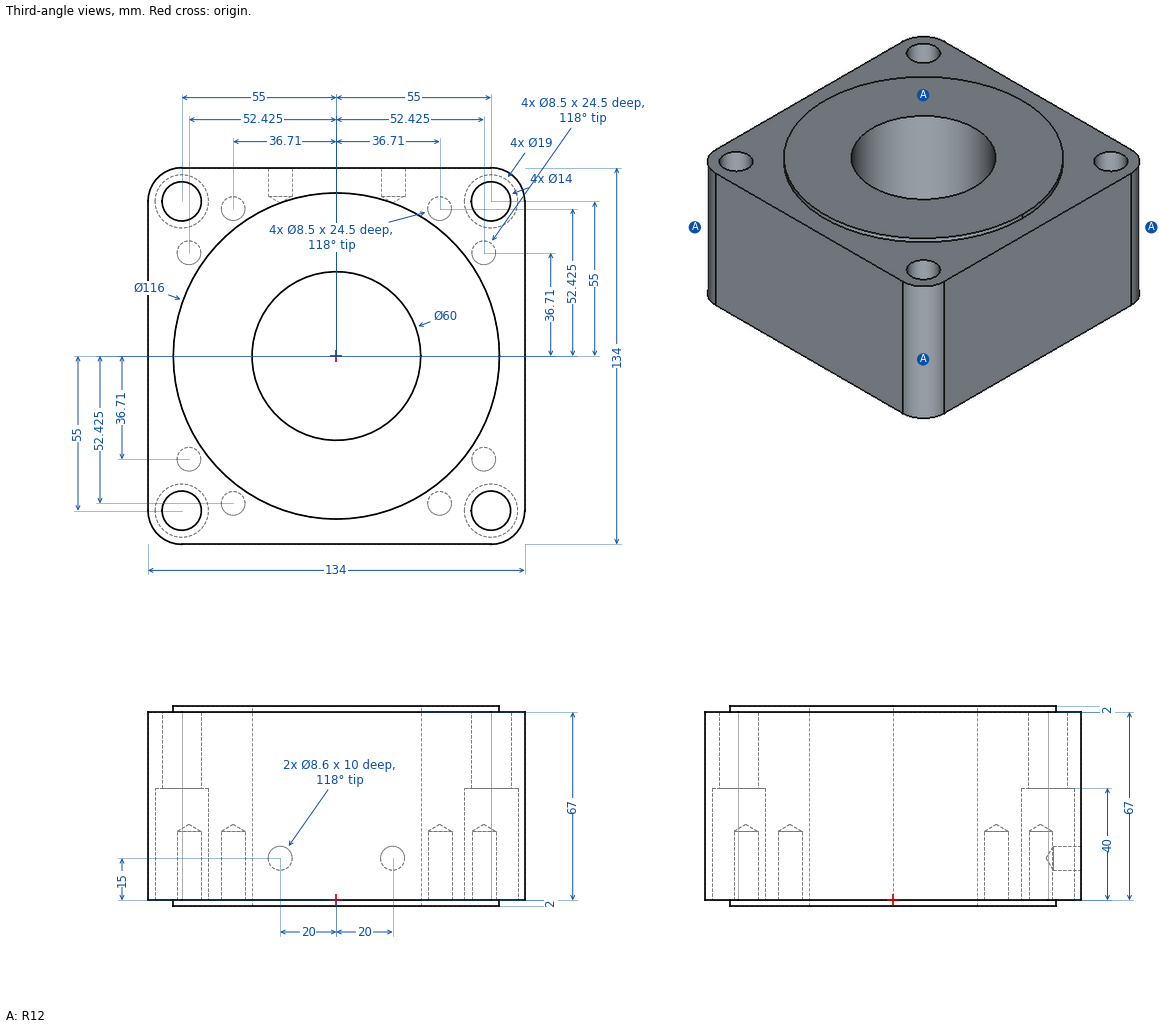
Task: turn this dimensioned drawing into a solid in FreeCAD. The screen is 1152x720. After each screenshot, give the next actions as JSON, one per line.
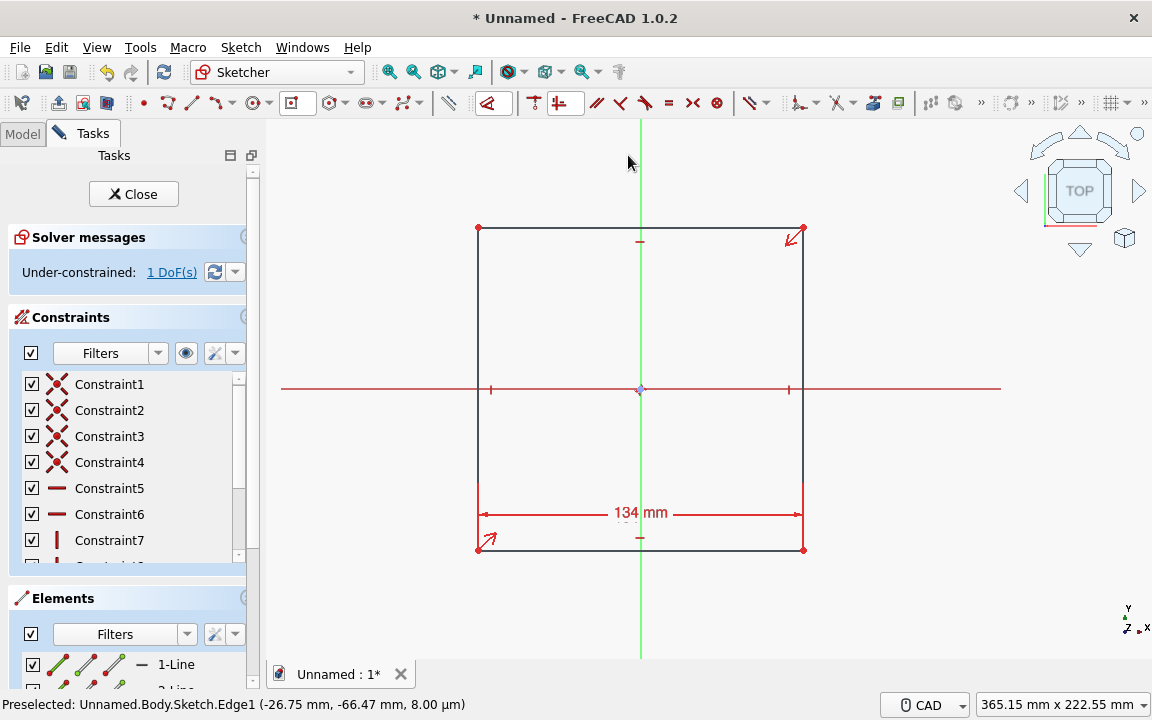
{"action": "left_click", "coordinate": [803, 454]}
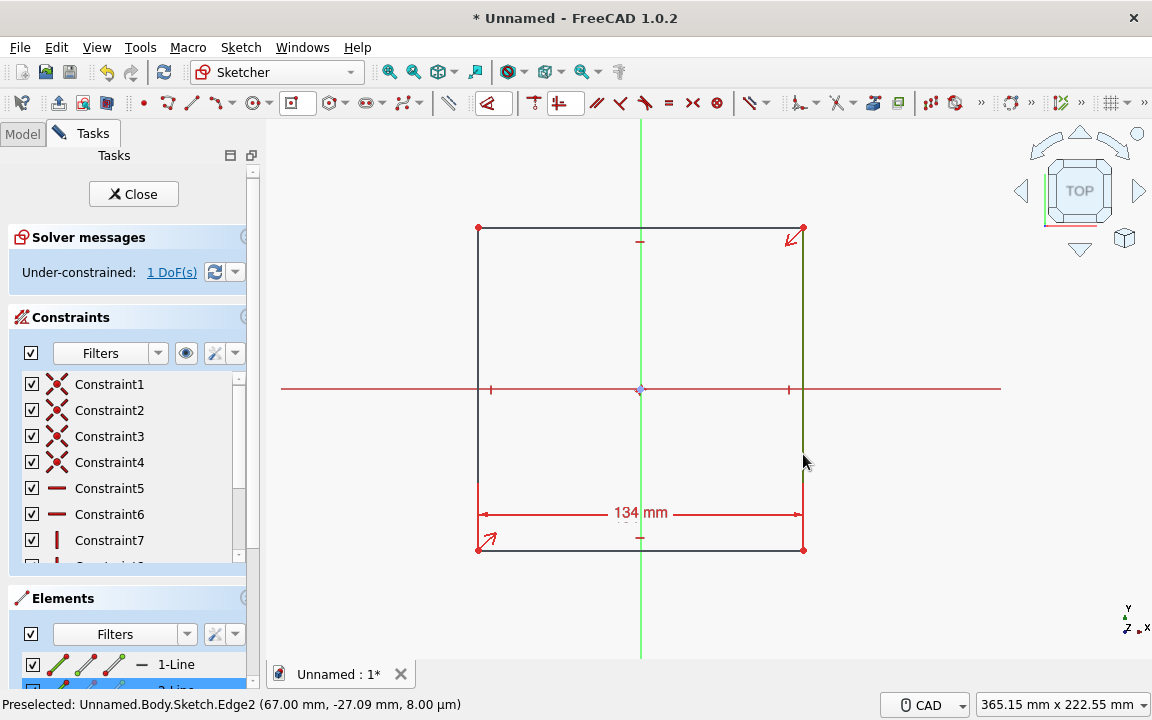
{"action": "left_click", "coordinate": [506, 104]}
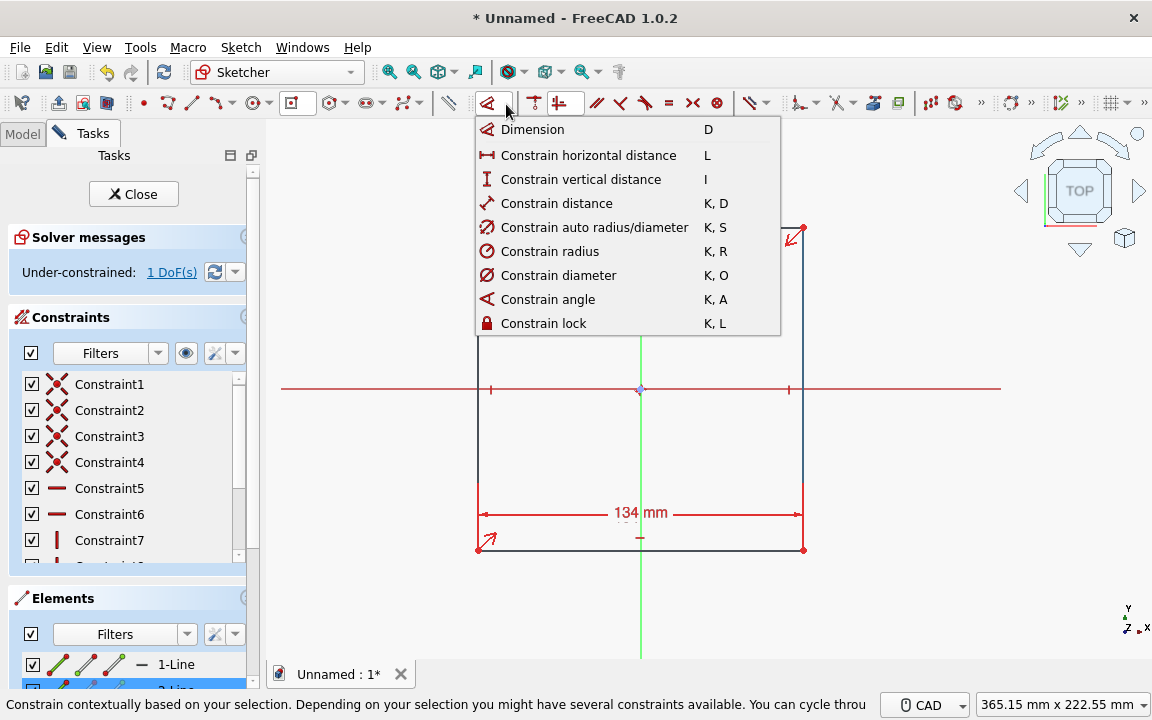
{"action": "left_click", "coordinate": [628, 179]}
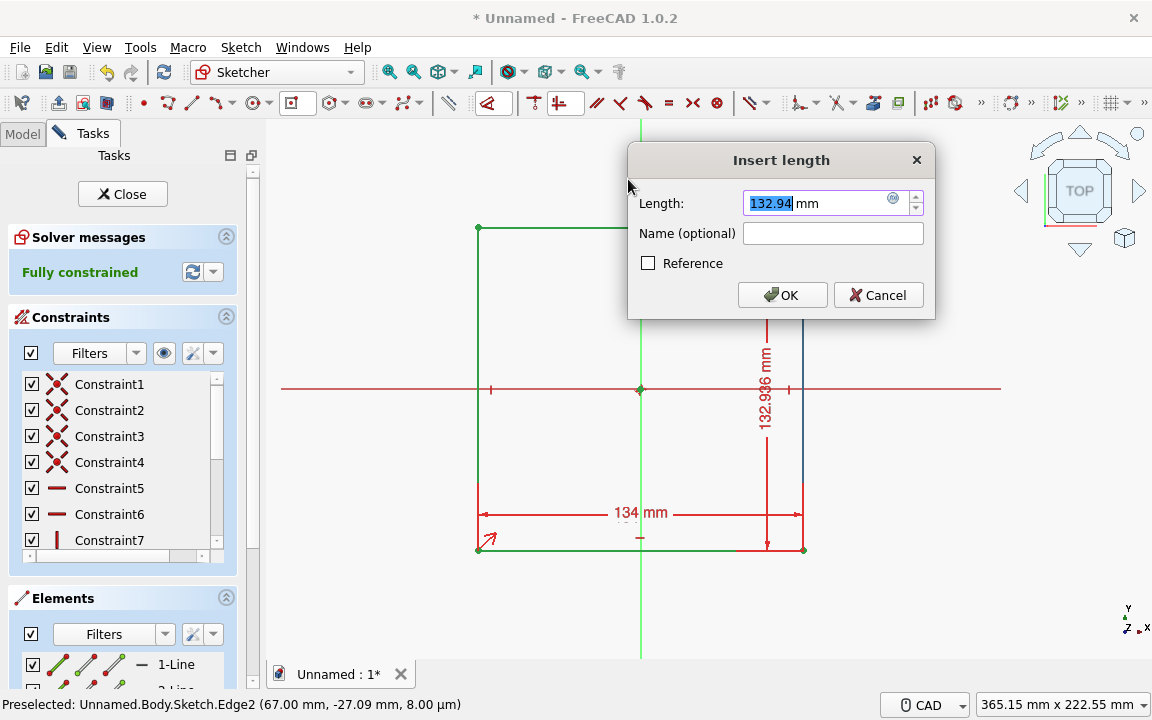
{"action": "type", "text": "134"}
{"action": "key", "text": "Return"}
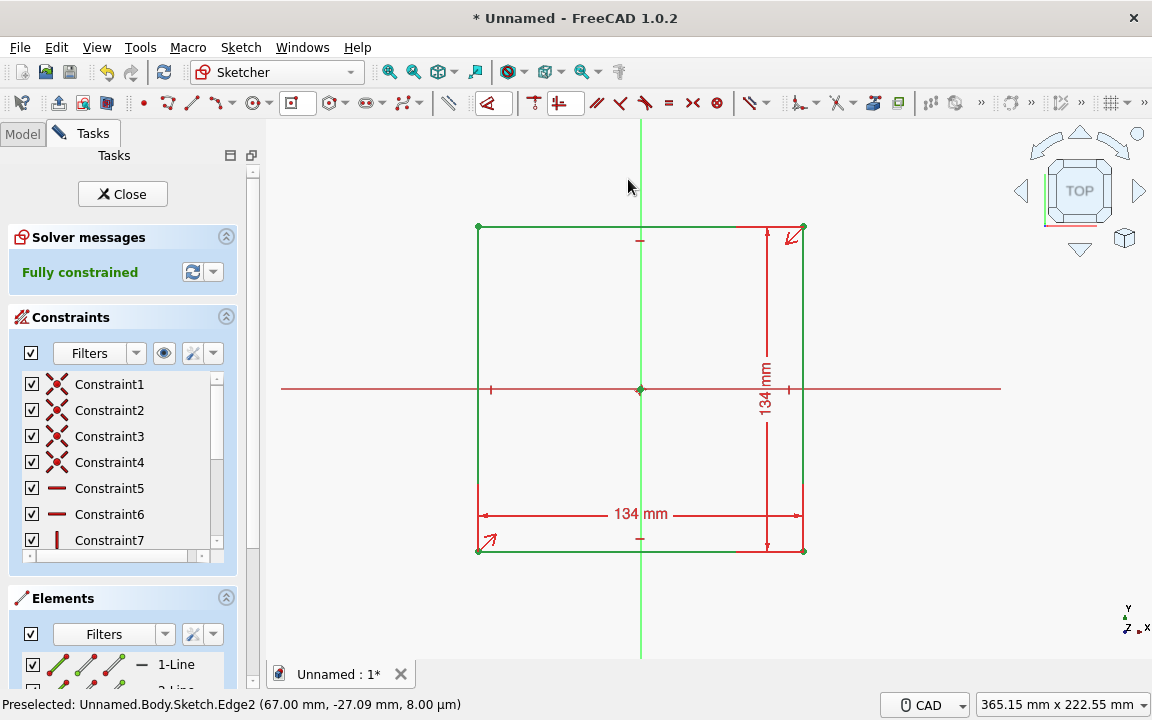
{"action": "left_click", "coordinate": [123, 194]}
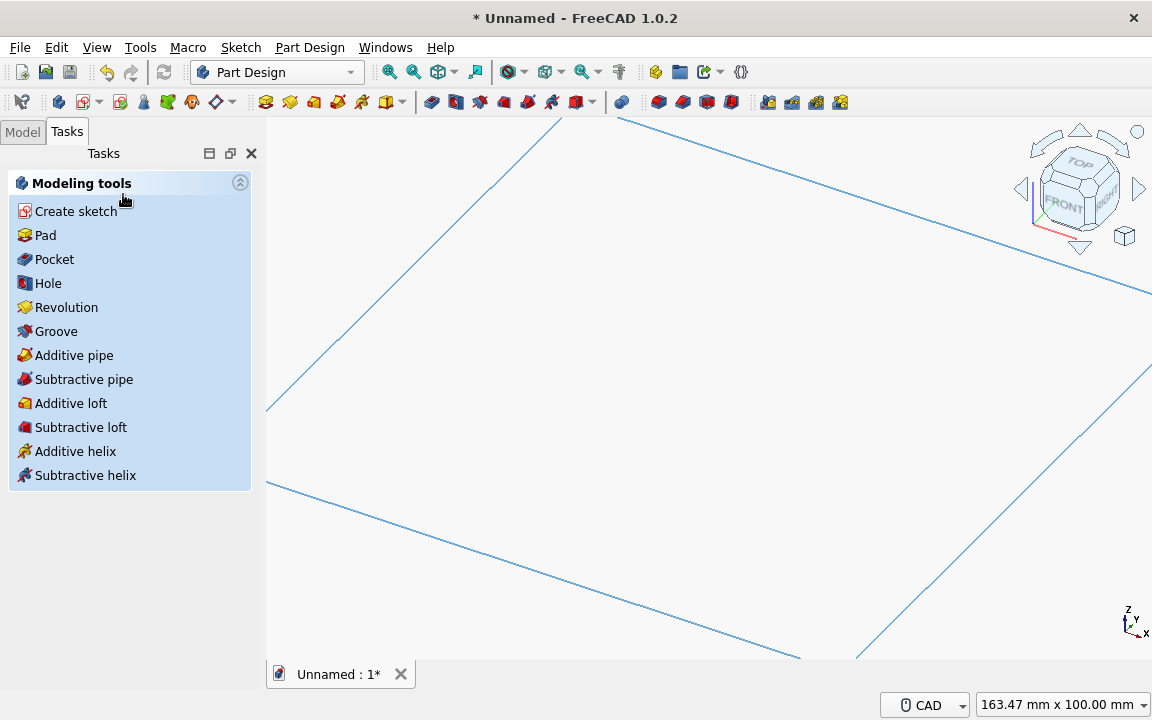
{"action": "left_click", "coordinate": [266, 102]}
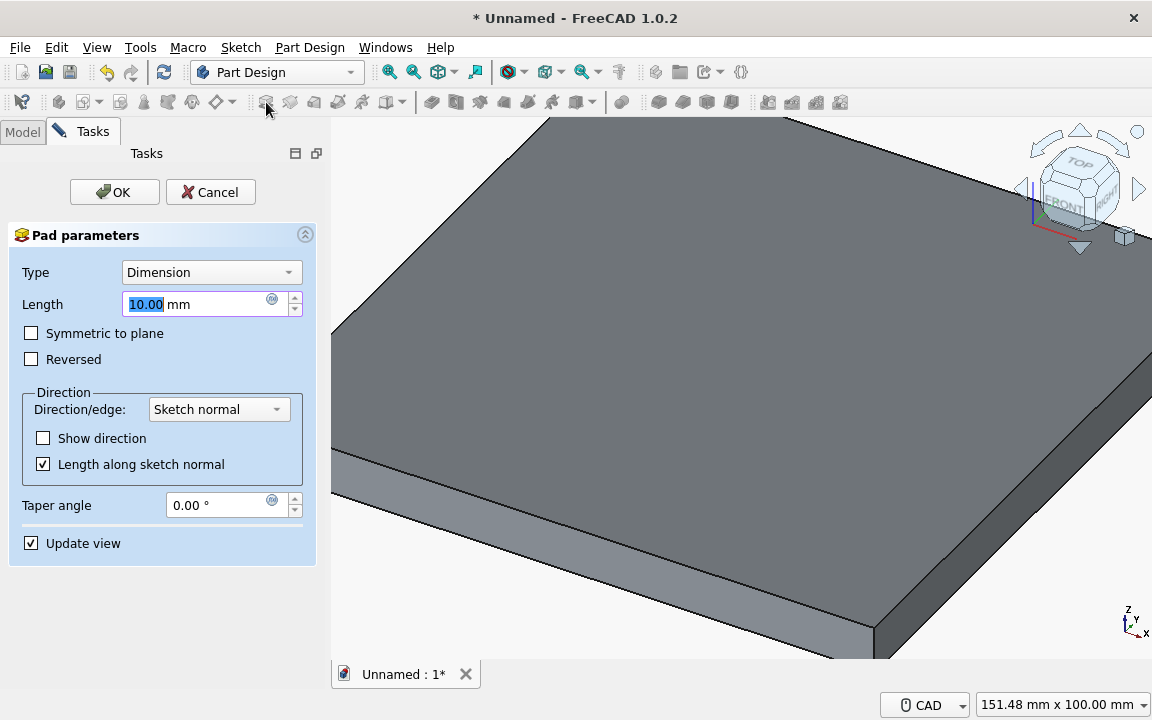
{"action": "type", "text": "67"}
{"action": "key", "text": "Tab"}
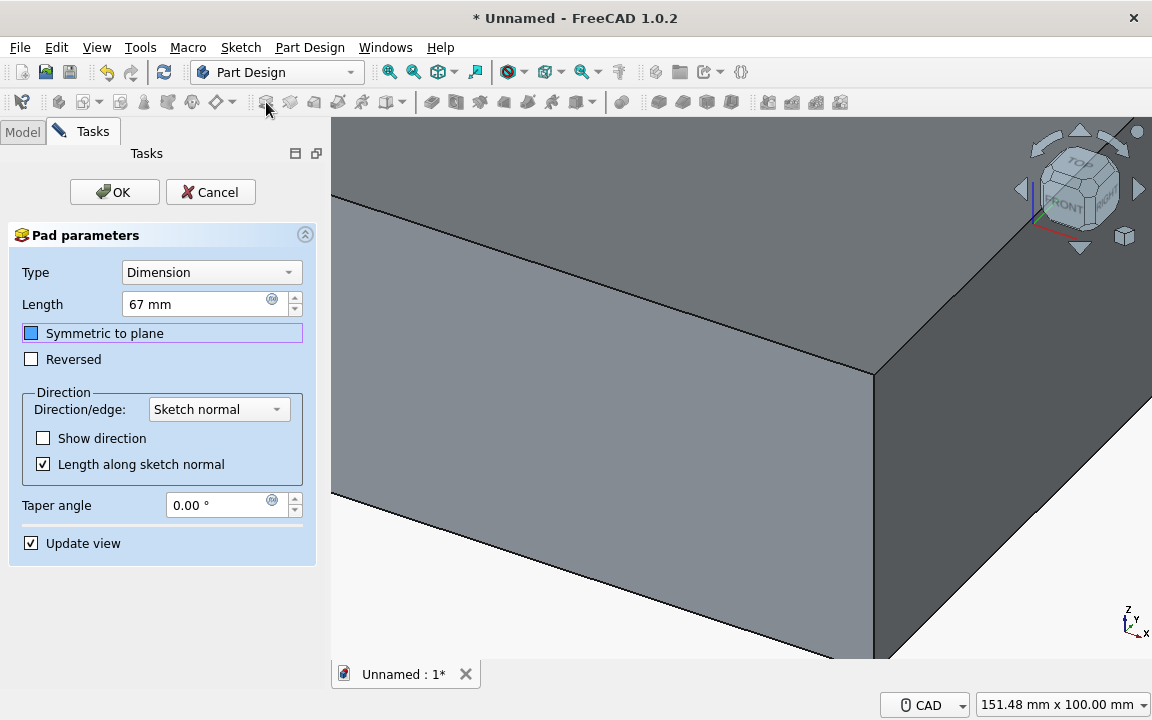
{"action": "left_click", "coordinate": [115, 192]}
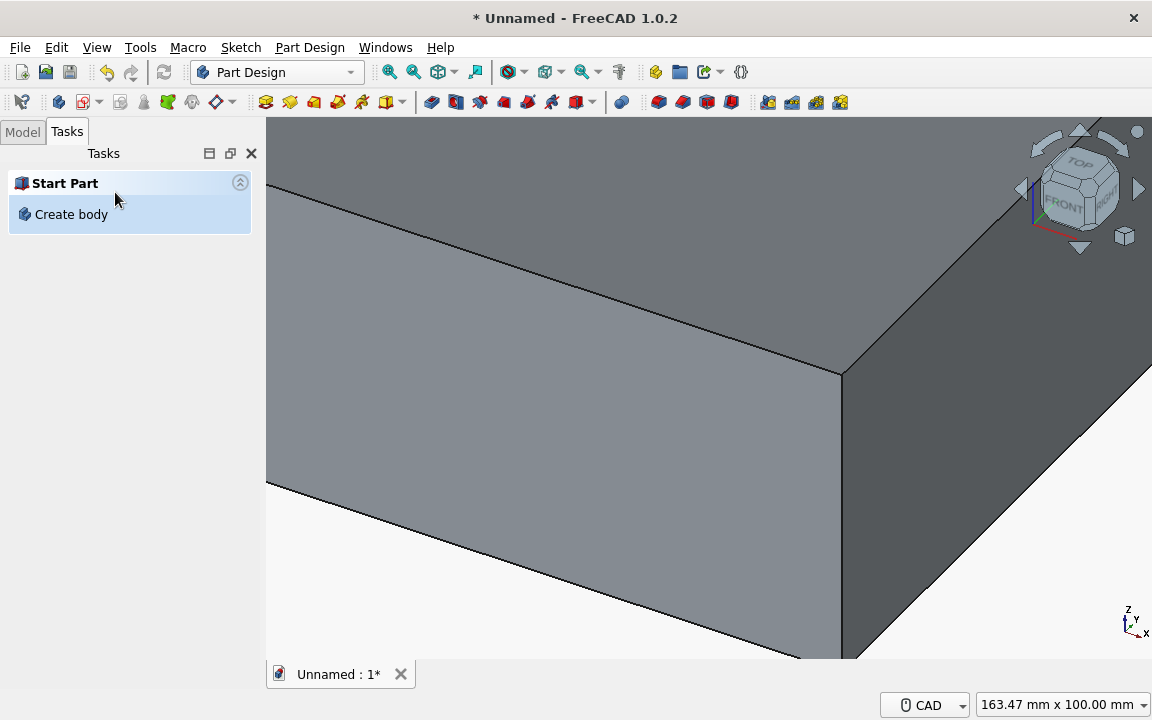
{"action": "left_click", "coordinate": [390, 72]}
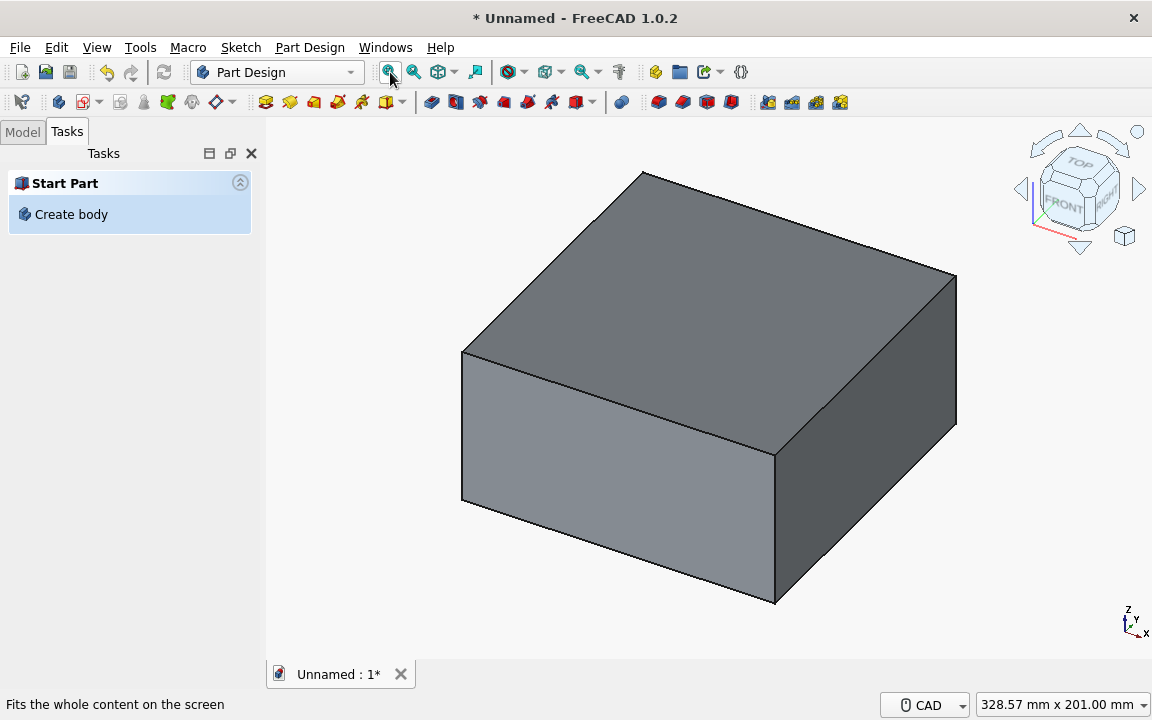
{"action": "left_click", "coordinate": [775, 529]}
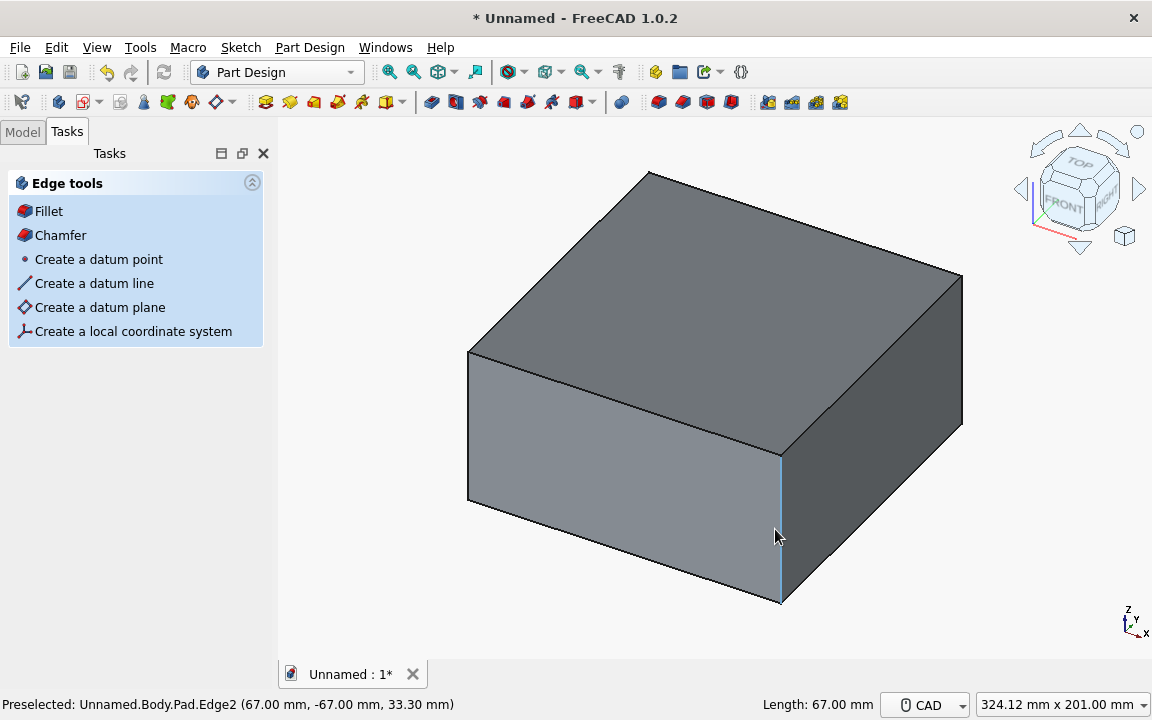
{"action": "key", "text": "0"}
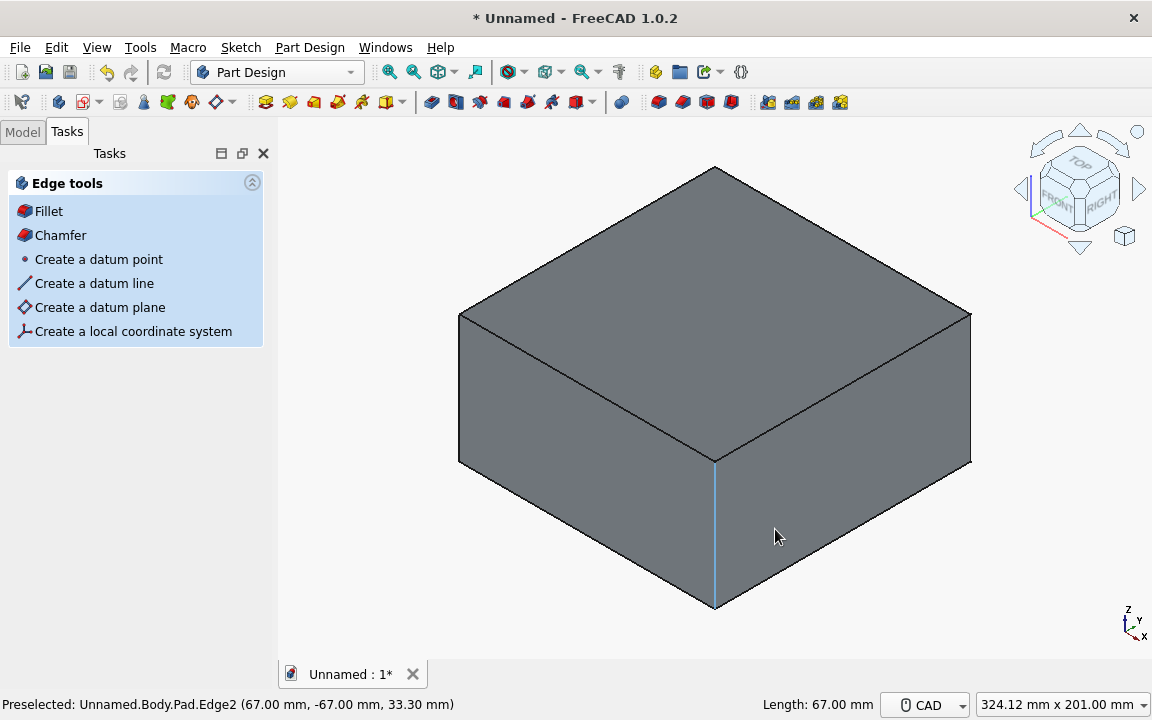
{"action": "key", "text": "2"}